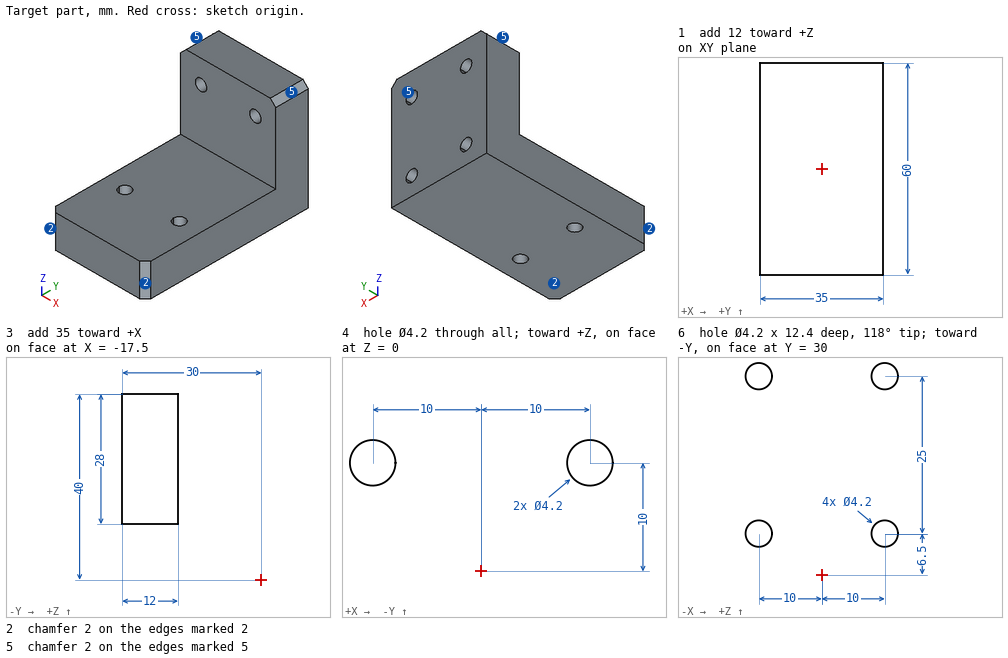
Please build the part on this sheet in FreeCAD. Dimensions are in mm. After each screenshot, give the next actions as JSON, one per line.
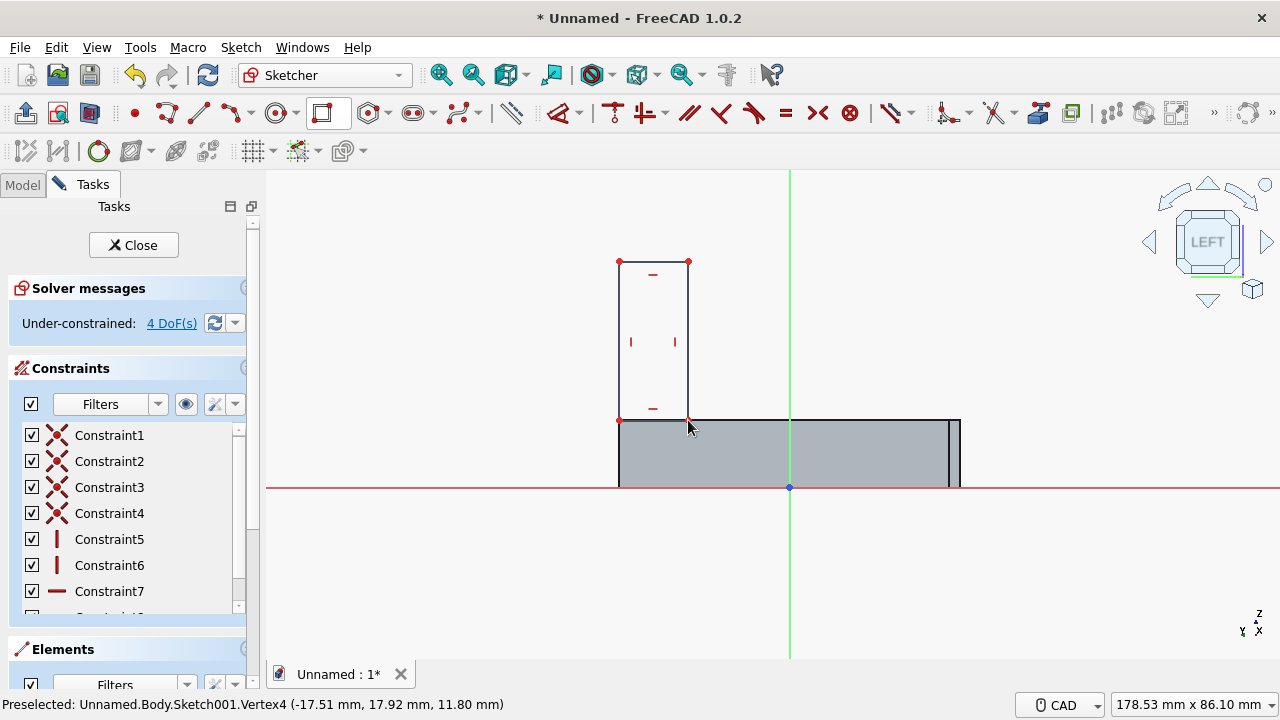
{"action": "left_click", "coordinate": [558, 114]}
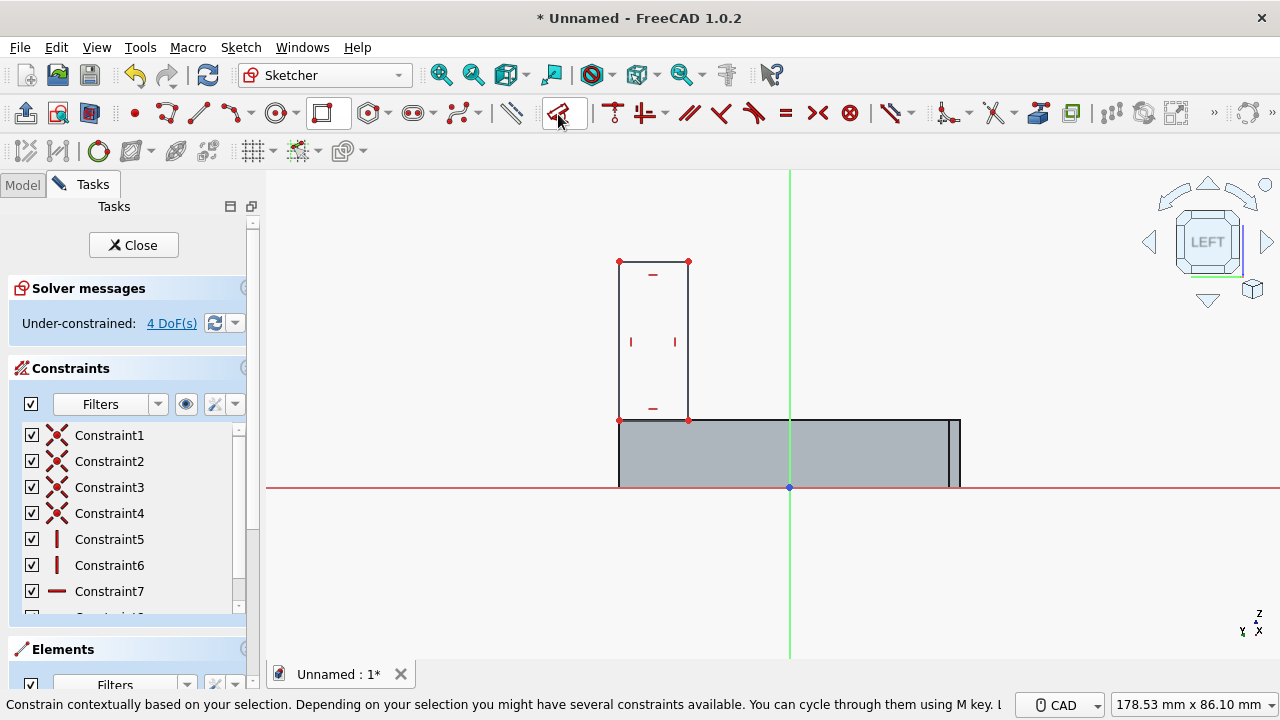
{"action": "left_click", "coordinate": [619, 310]}
{"action": "left_click", "coordinate": [585, 342]}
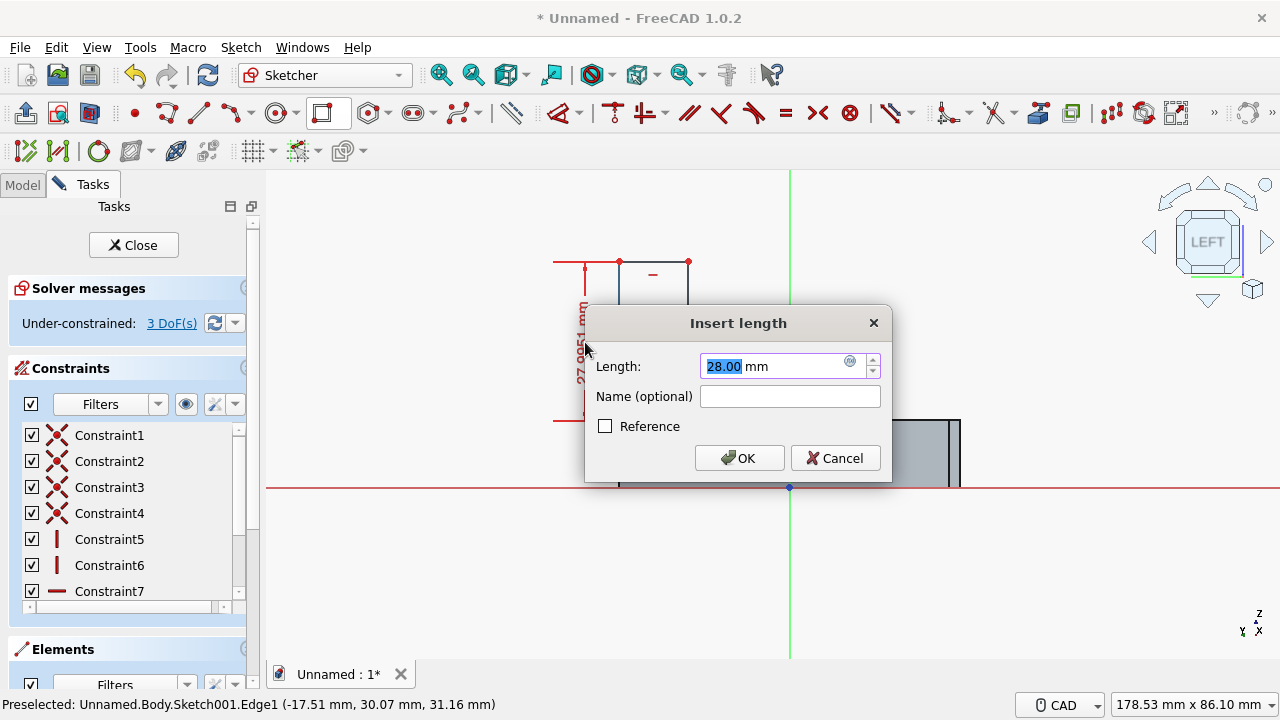
{"action": "type", "text": "28"}
{"action": "key", "text": "Return"}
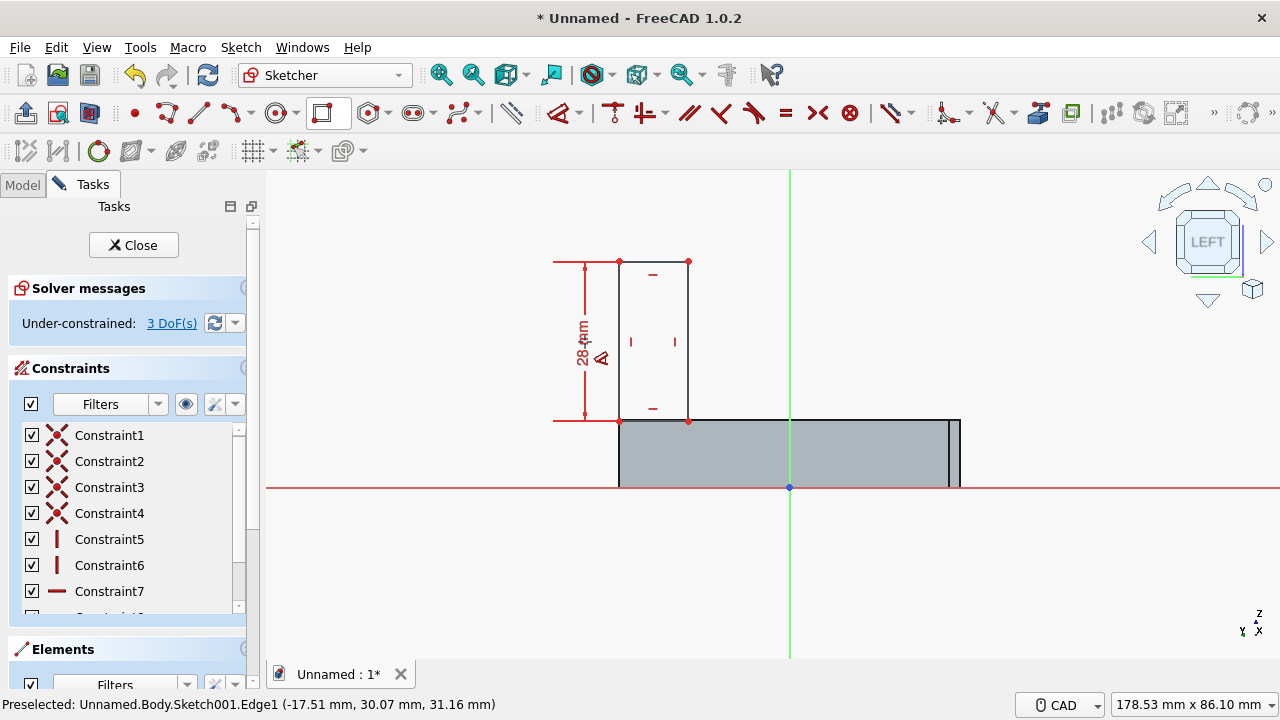
{"action": "left_click", "coordinate": [640, 421]}
{"action": "left_click", "coordinate": [654, 455]}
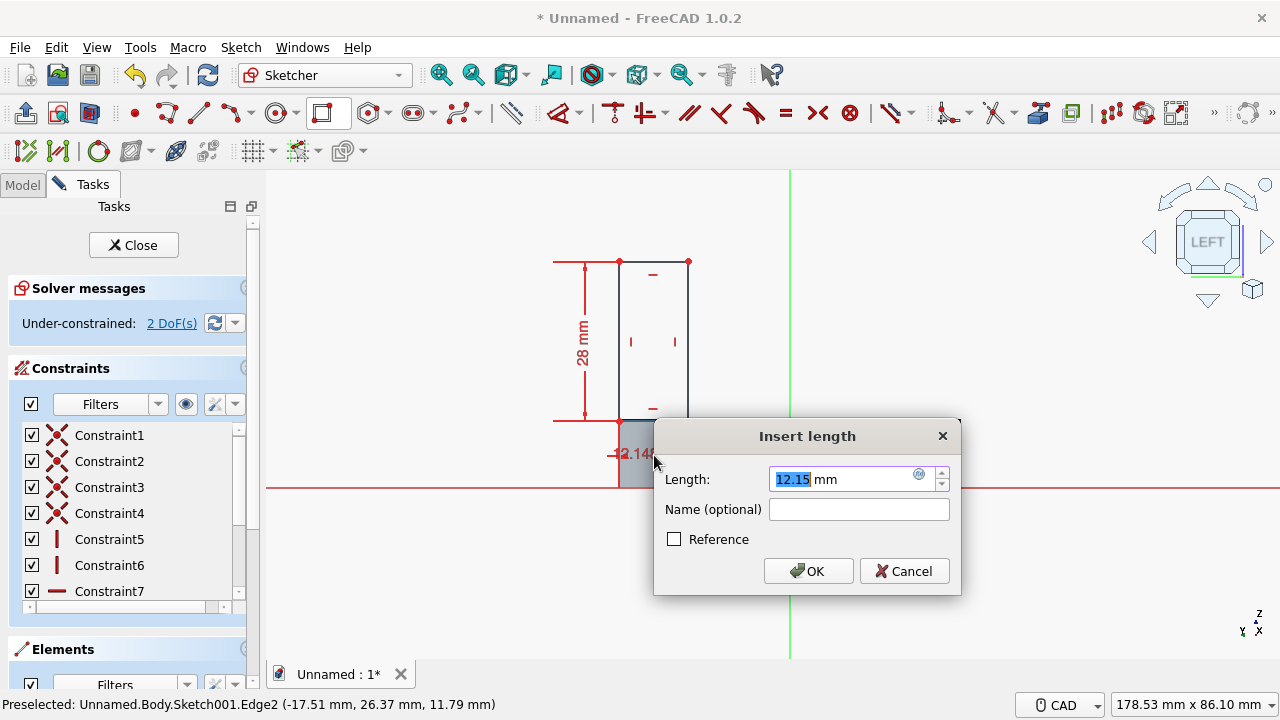
{"action": "type", "text": "12"}
{"action": "key", "text": "Return"}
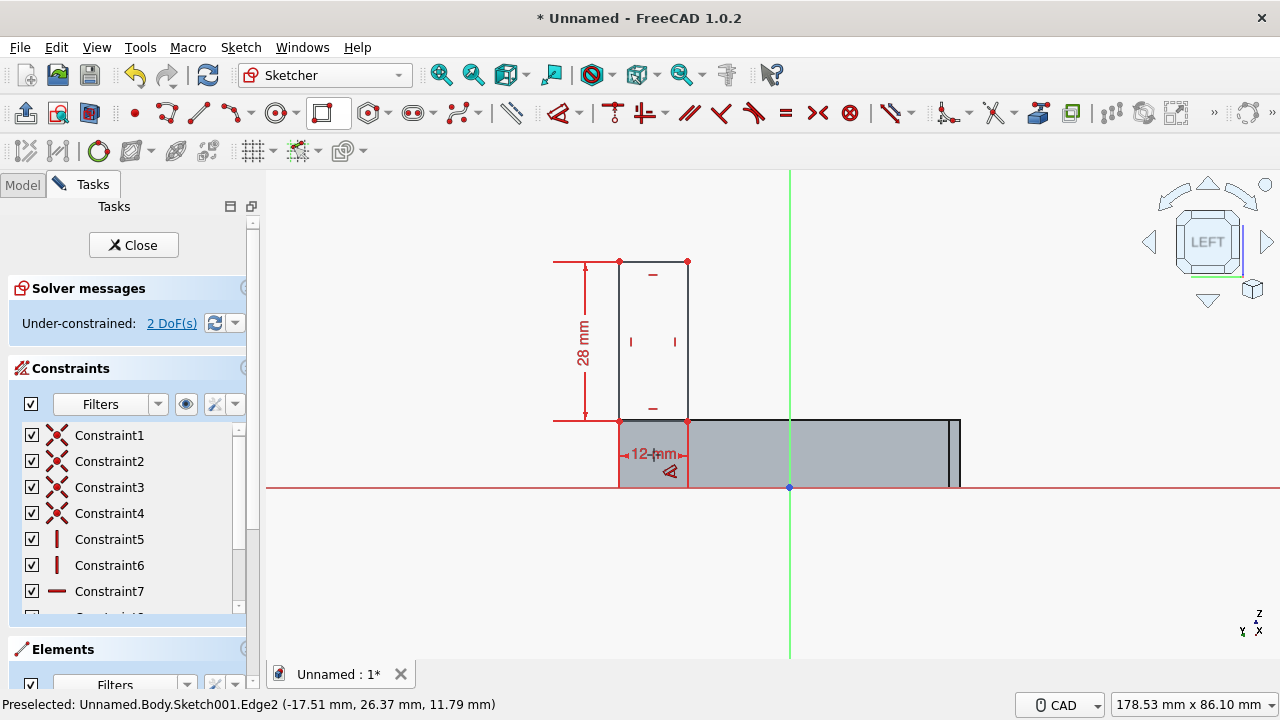
{"action": "left_click", "coordinate": [619, 262]}
{"action": "left_click", "coordinate": [705, 522]}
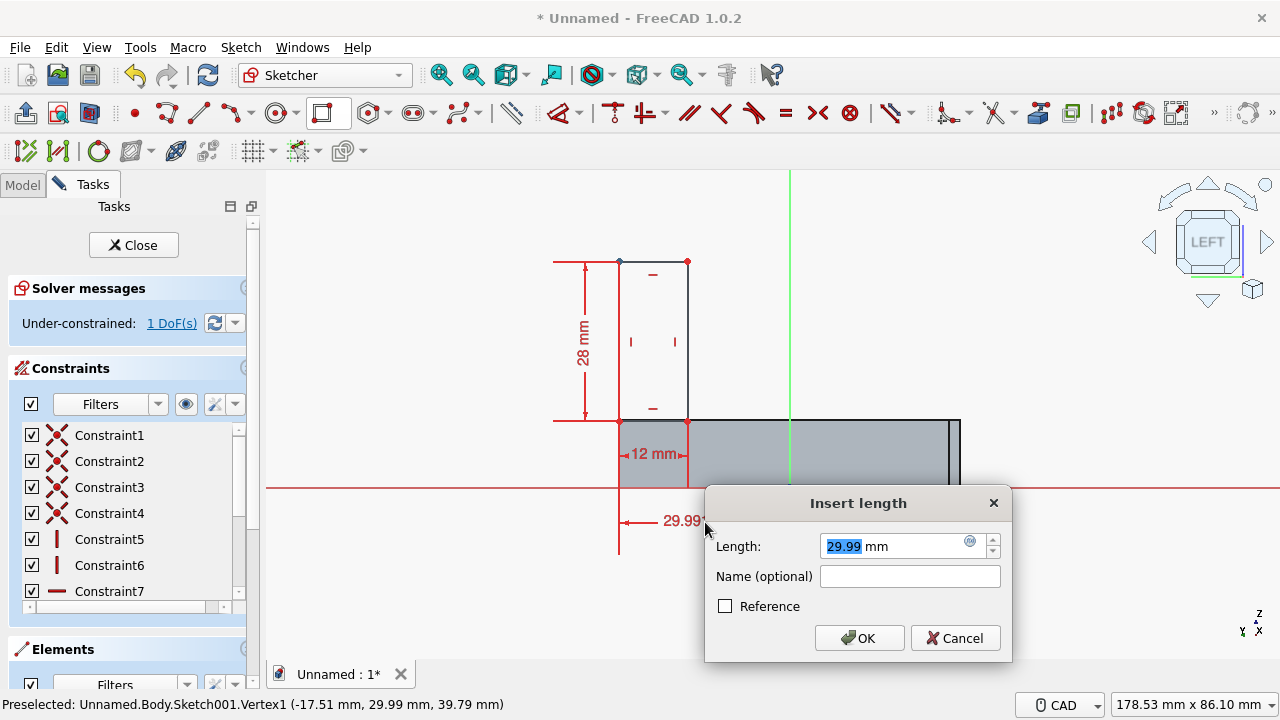
{"action": "type", "text": "30"}
{"action": "key", "text": "Return"}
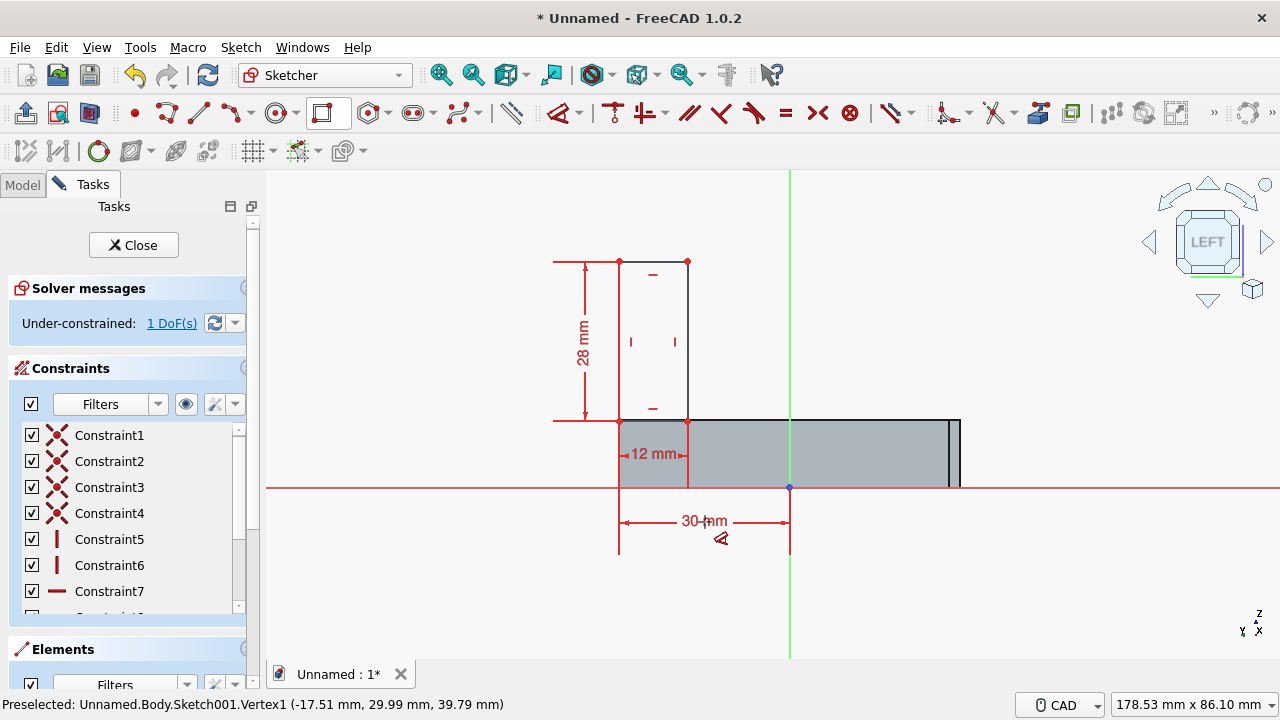
{"action": "left_click", "coordinate": [619, 262]}
{"action": "left_click", "coordinate": [824, 375]}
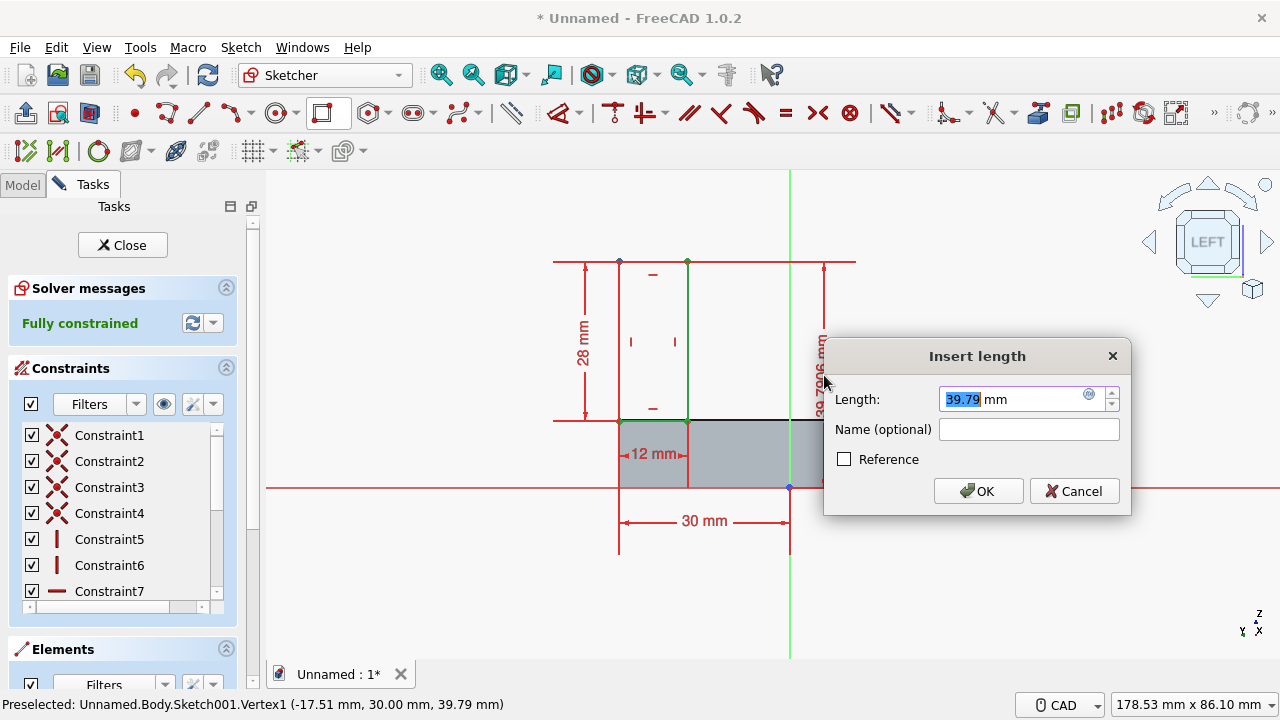
{"action": "type", "text": "40"}
{"action": "key", "text": "Return"}
{"action": "key", "text": "Escape"}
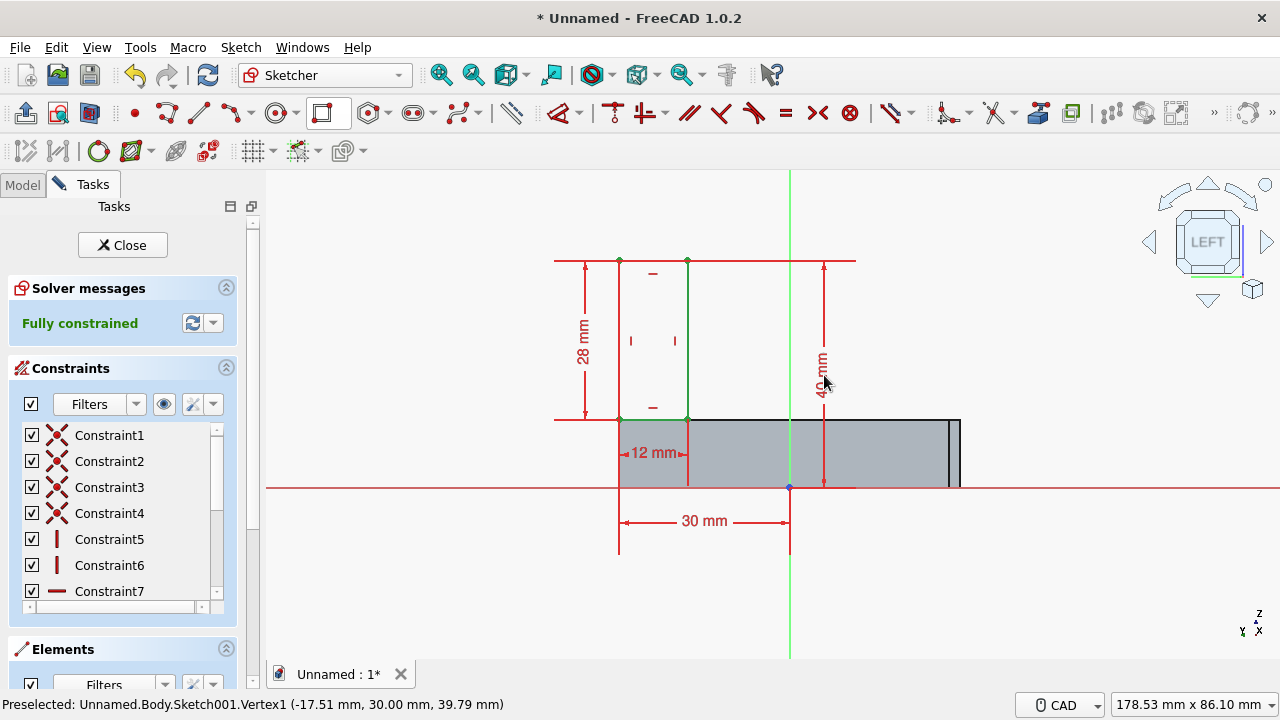
{"action": "left_click", "coordinate": [123, 245]}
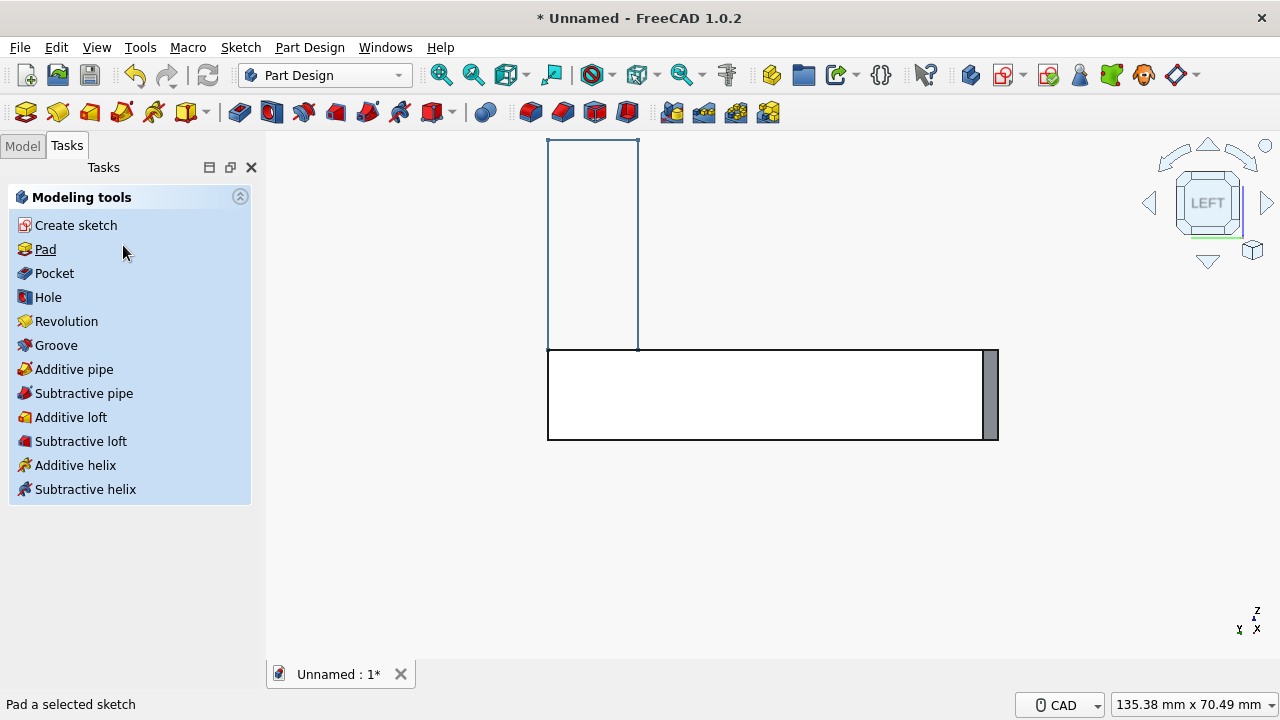
{"action": "left_click", "coordinate": [26, 112]}